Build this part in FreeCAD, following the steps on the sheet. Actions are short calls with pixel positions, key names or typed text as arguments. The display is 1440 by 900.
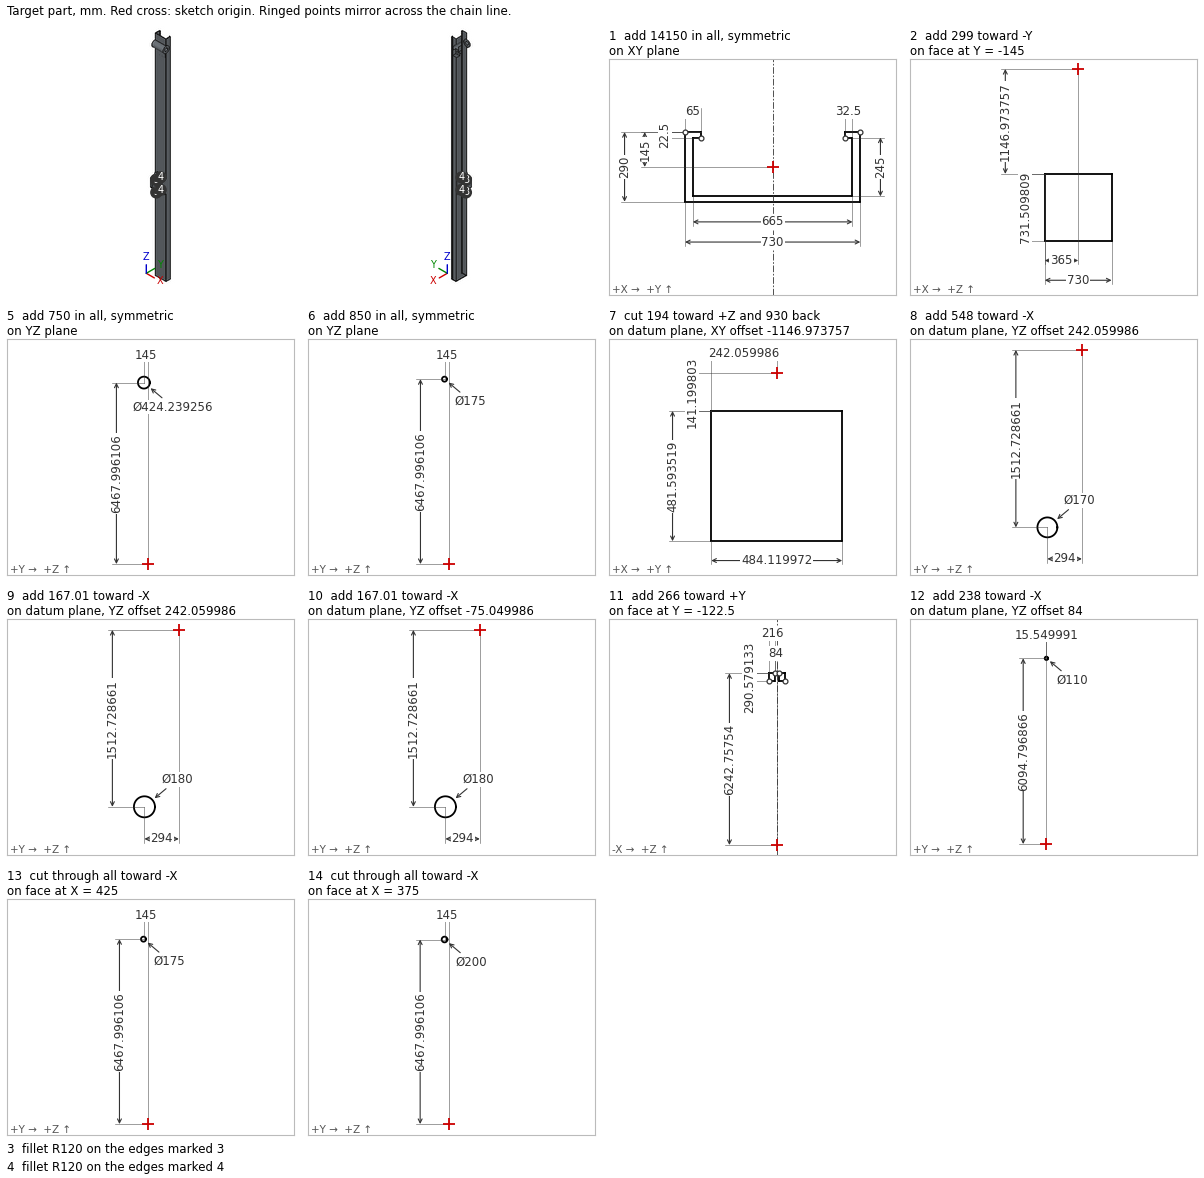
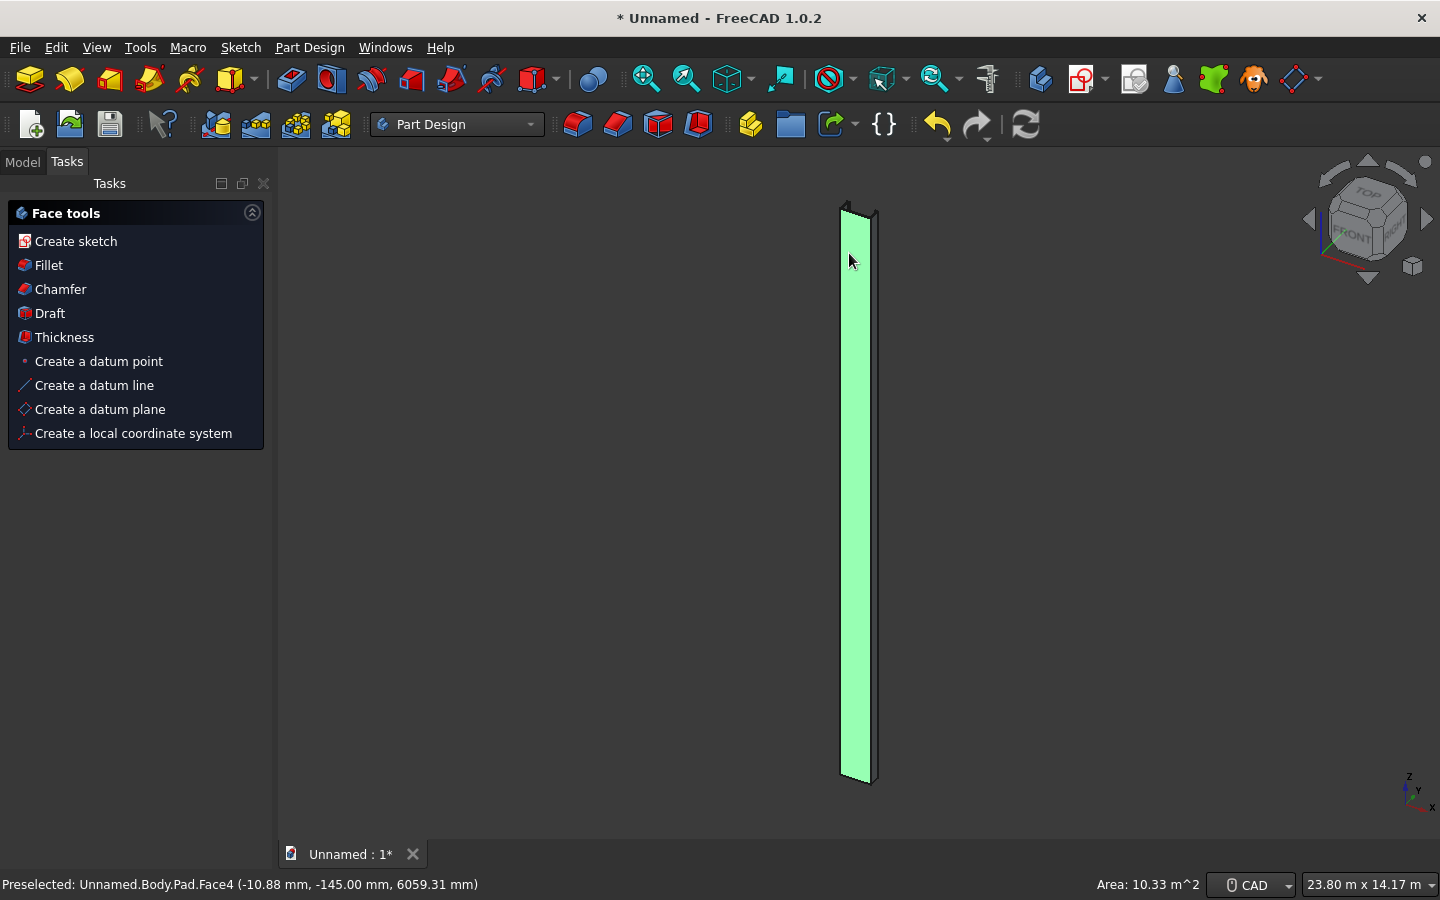
click(1082, 80)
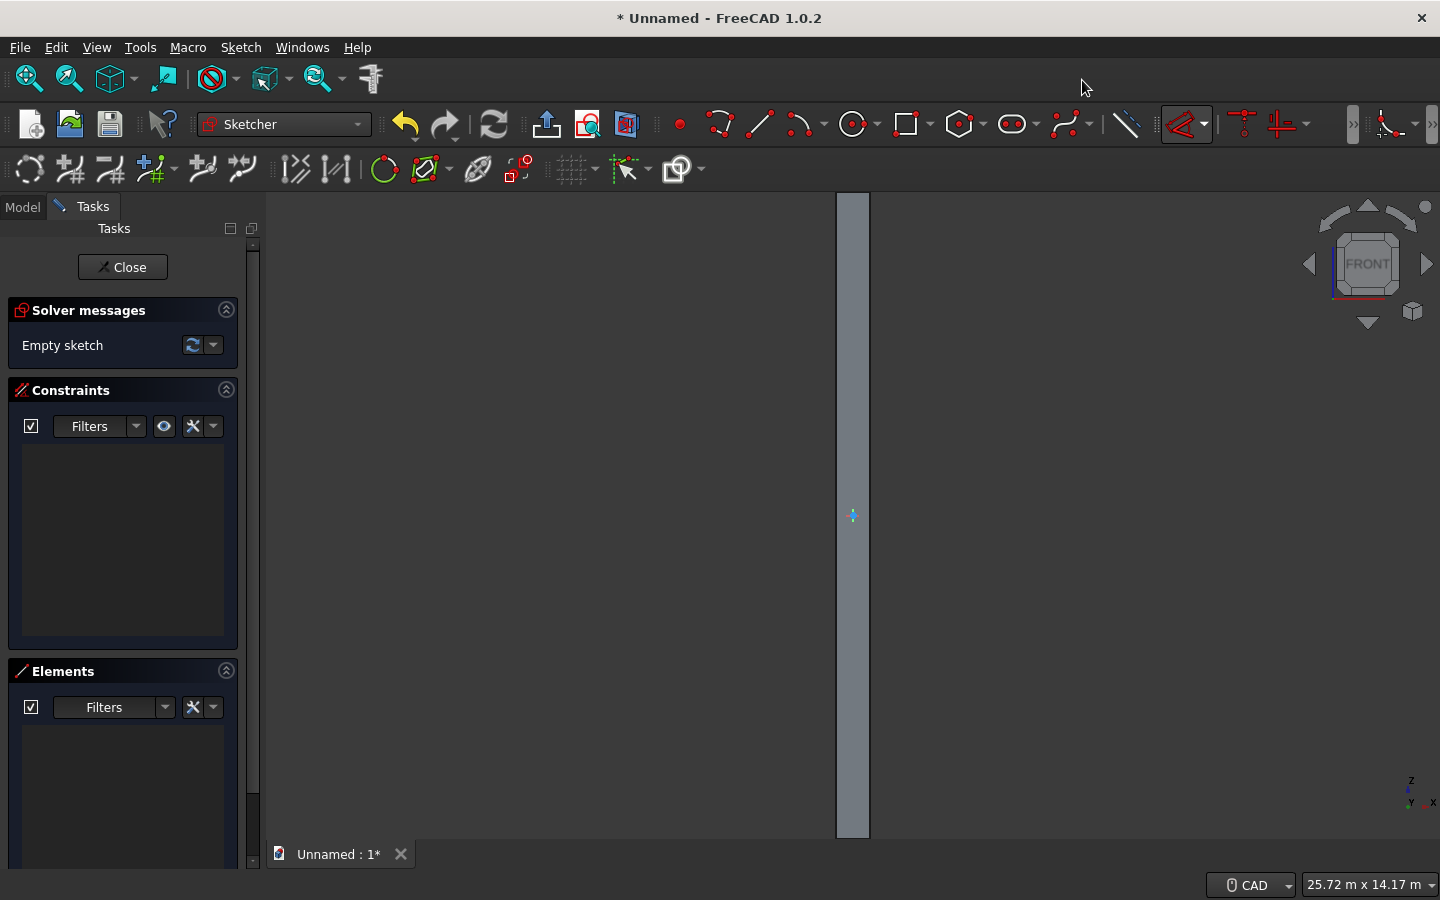
scroll(858, 590, up, 13)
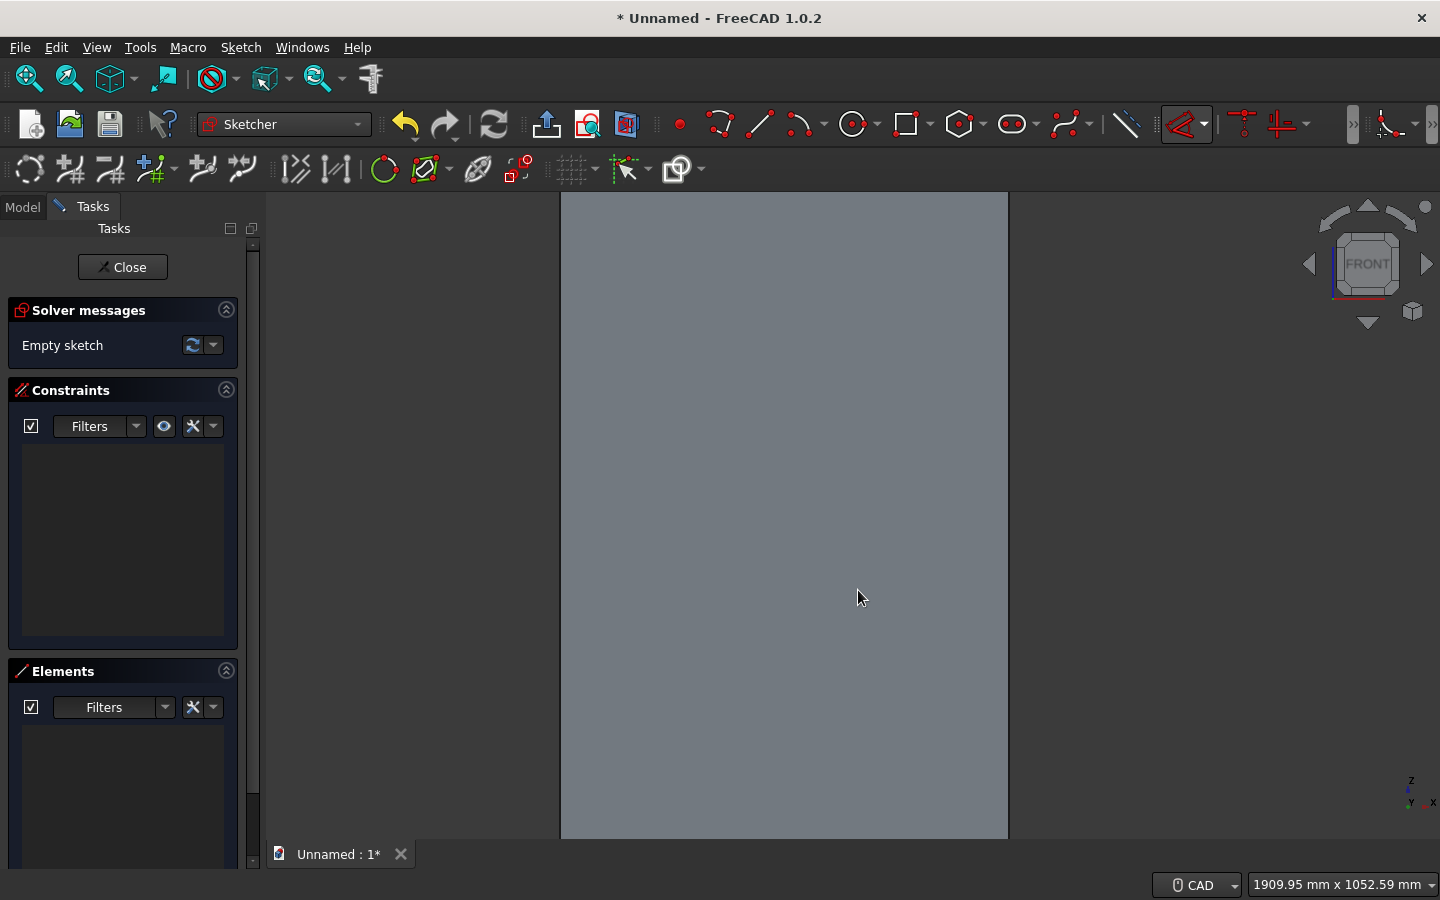
key(g)
key(r)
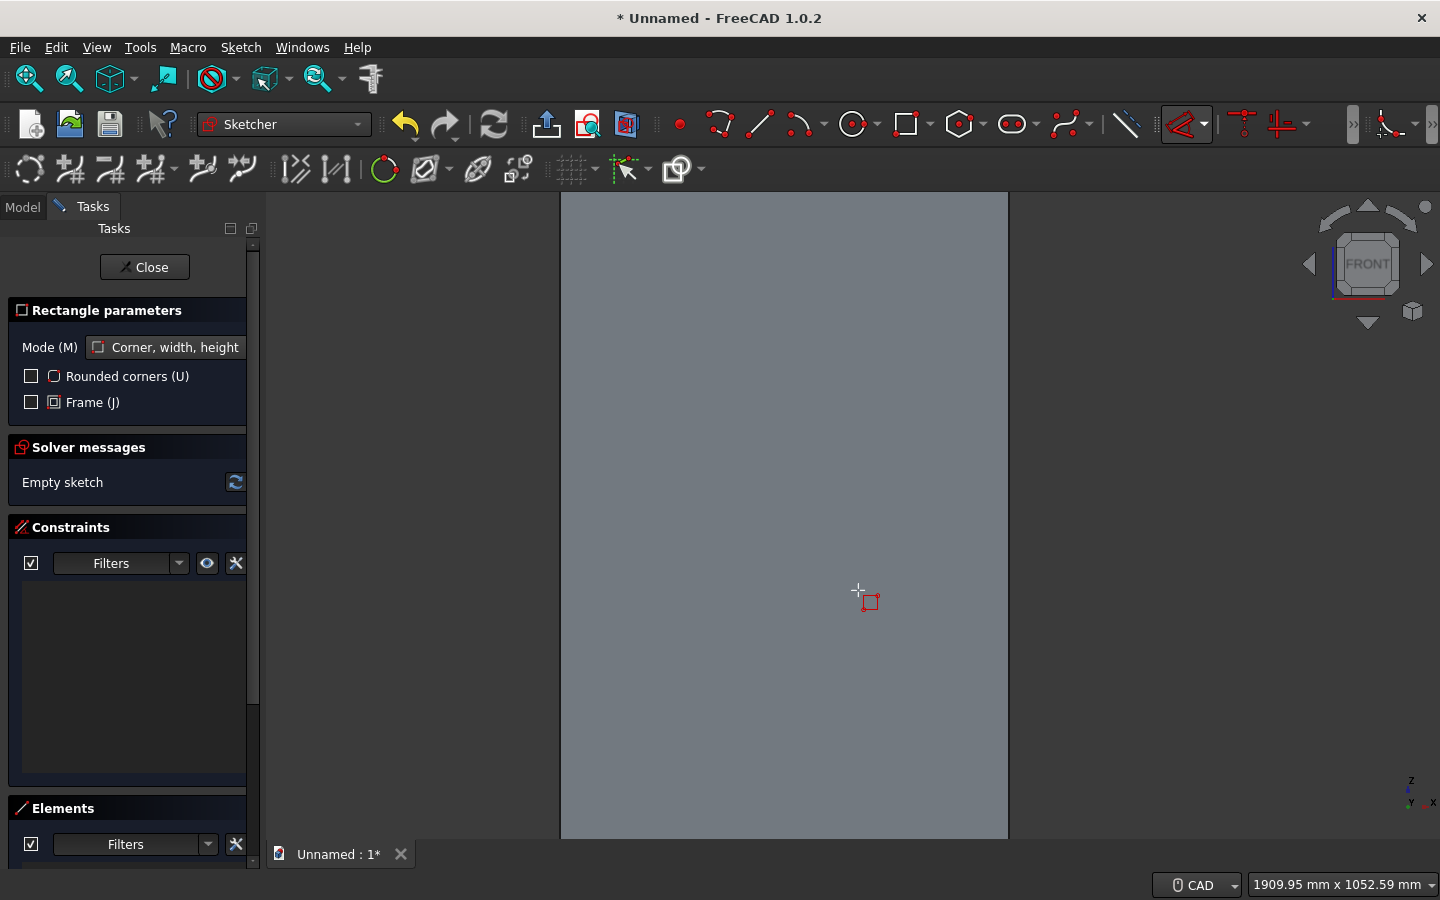
click(560, 284)
click(1009, 734)
key(Escape)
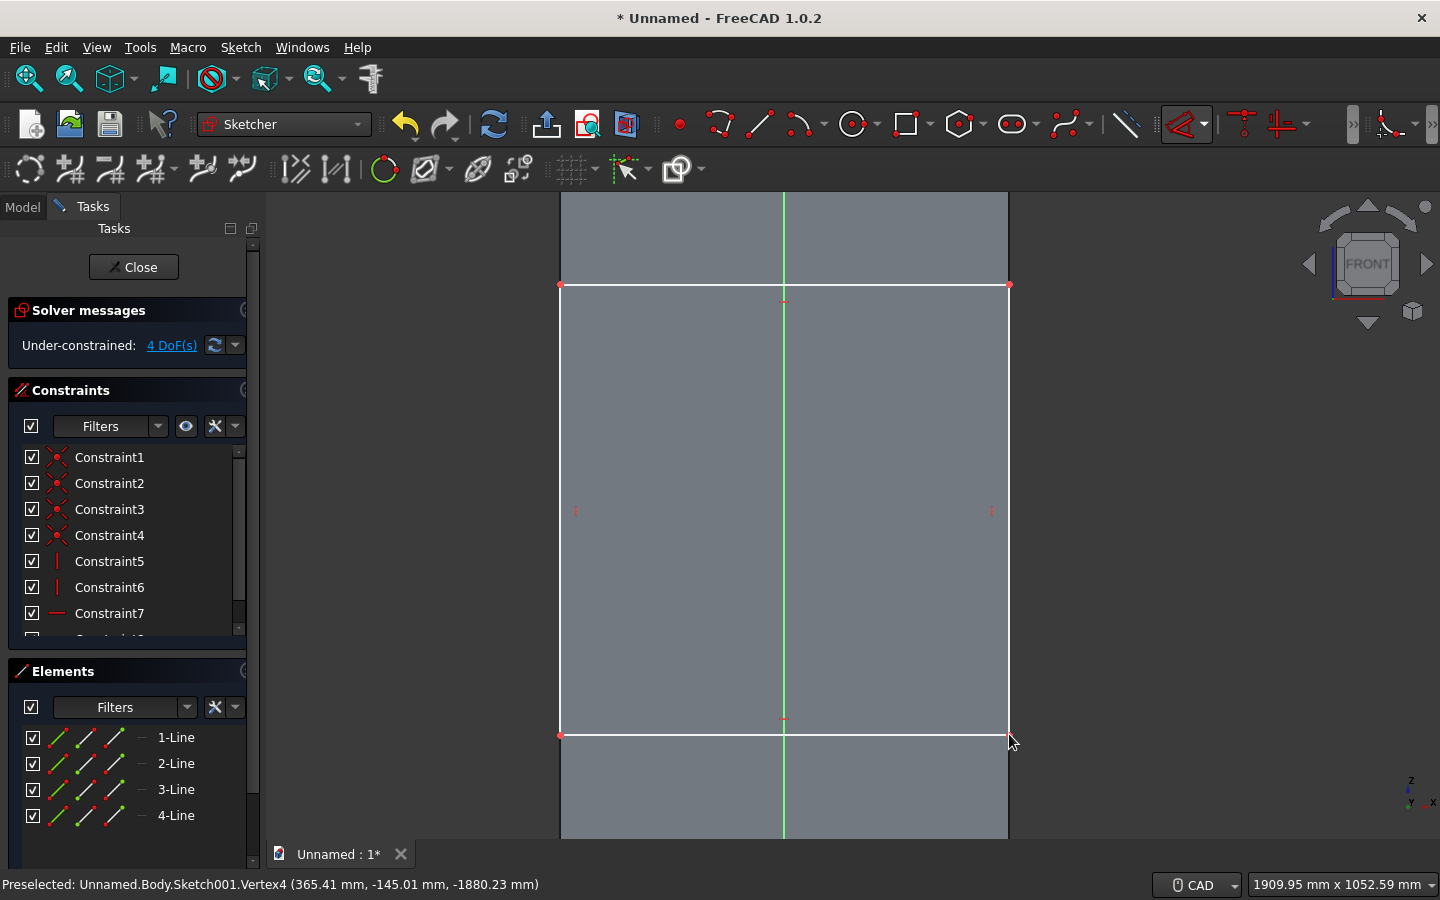
click(695, 735)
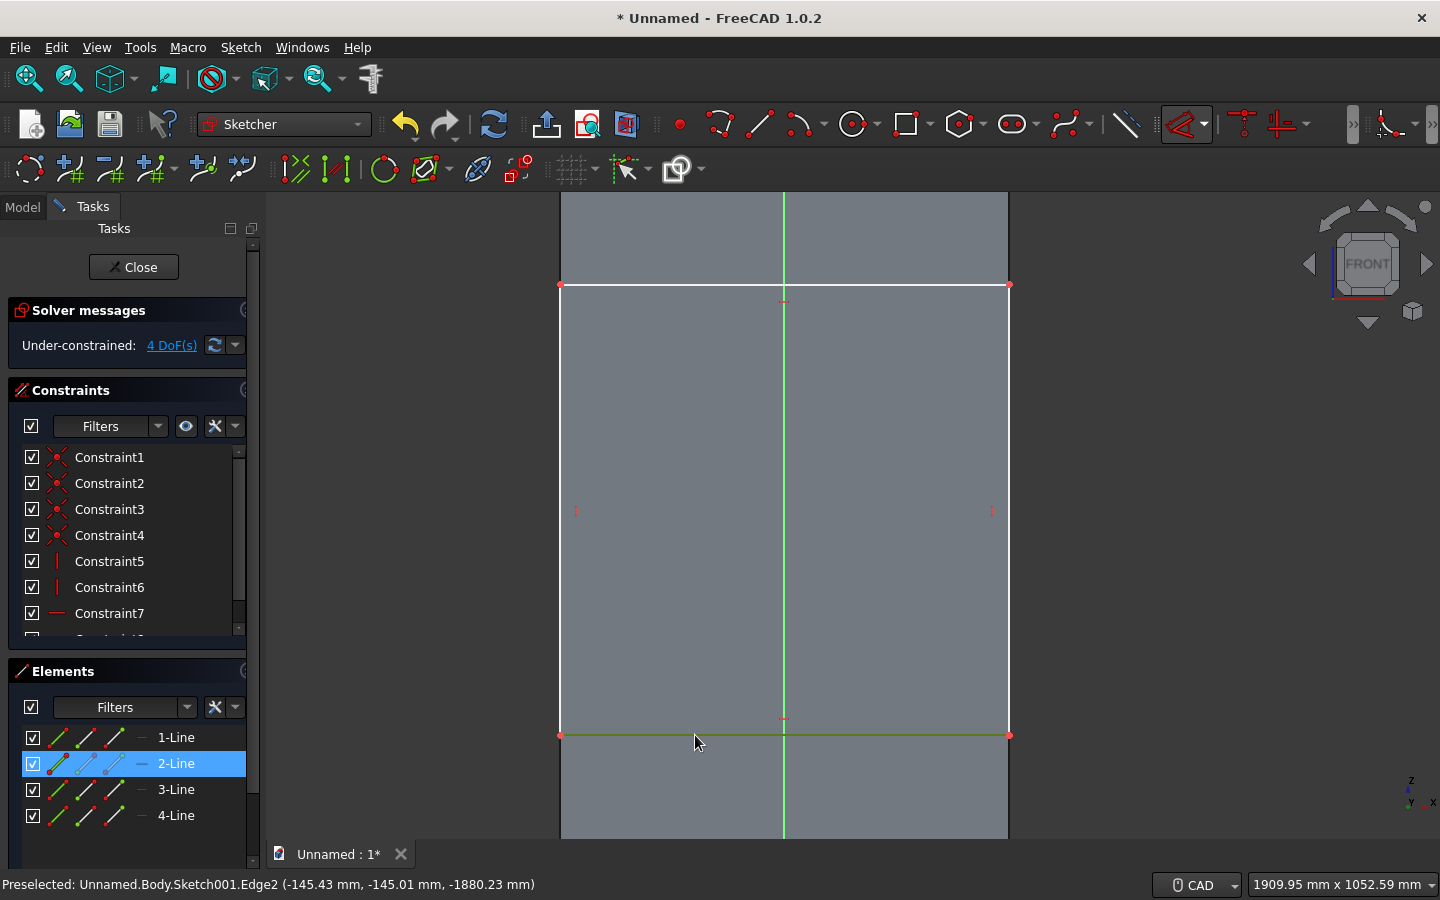
click(1206, 124)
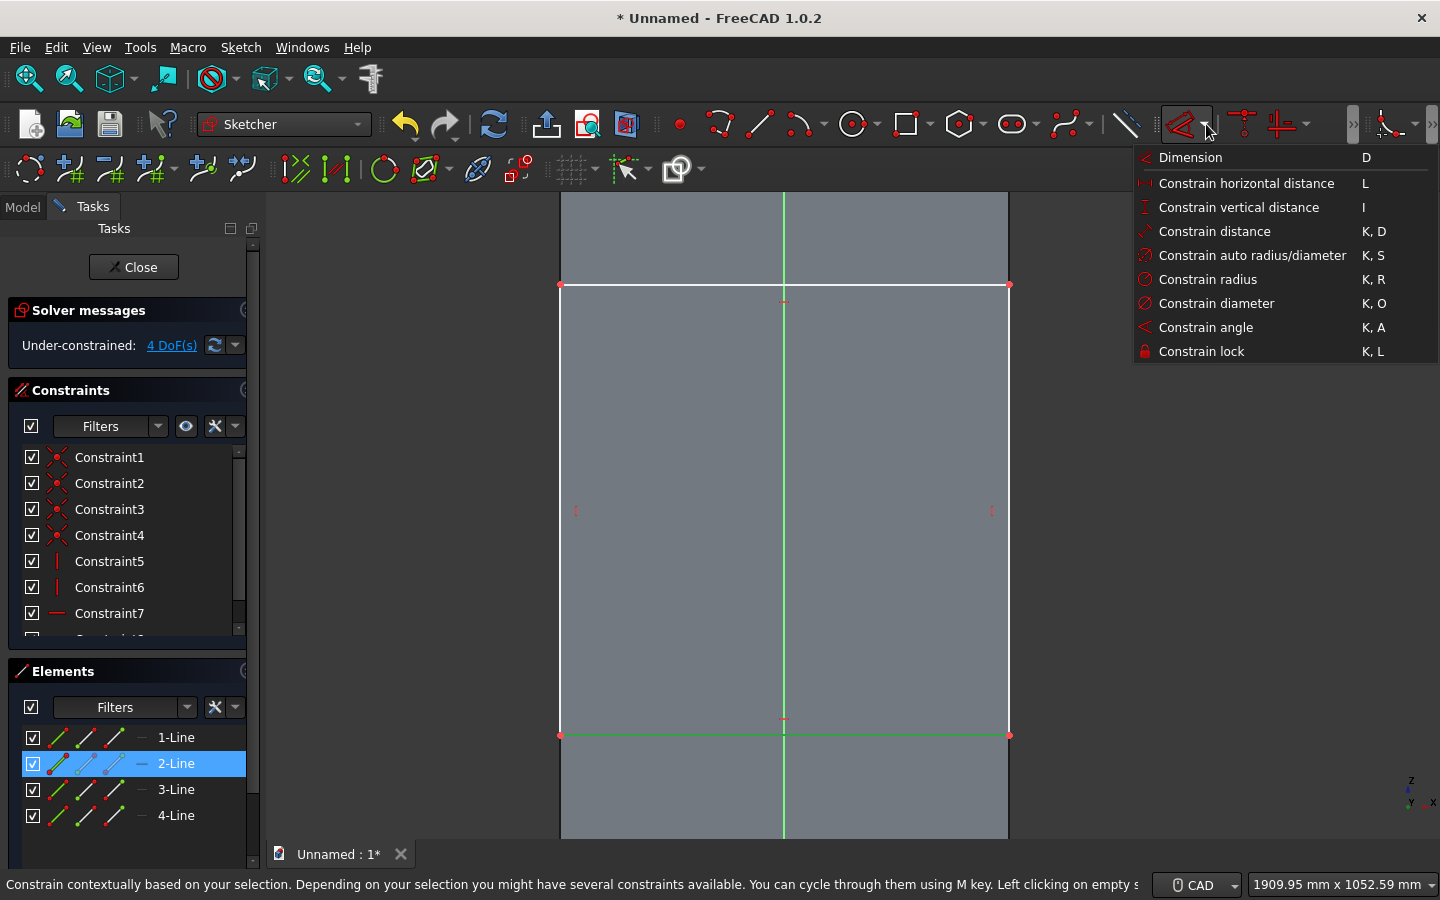
click(1286, 183)